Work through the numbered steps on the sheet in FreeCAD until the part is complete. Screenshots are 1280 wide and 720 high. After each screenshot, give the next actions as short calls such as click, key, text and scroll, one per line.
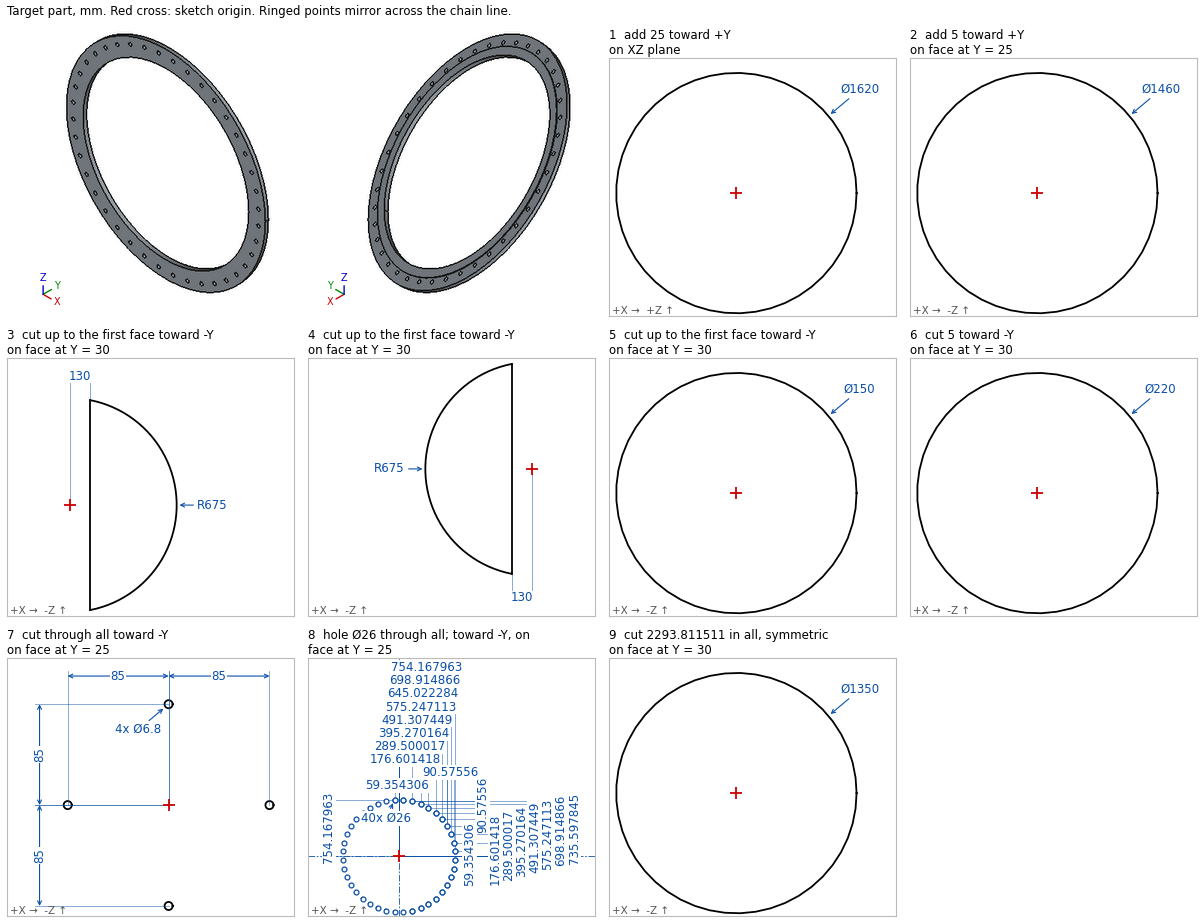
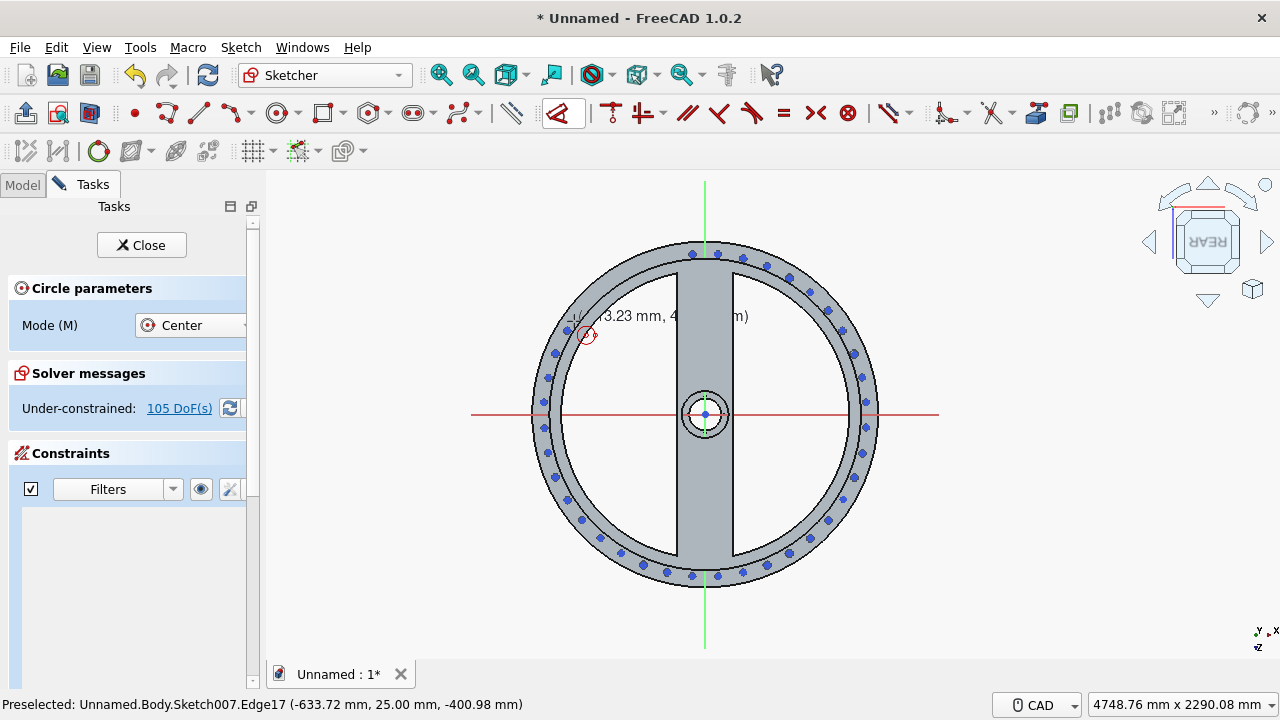
click(582, 310)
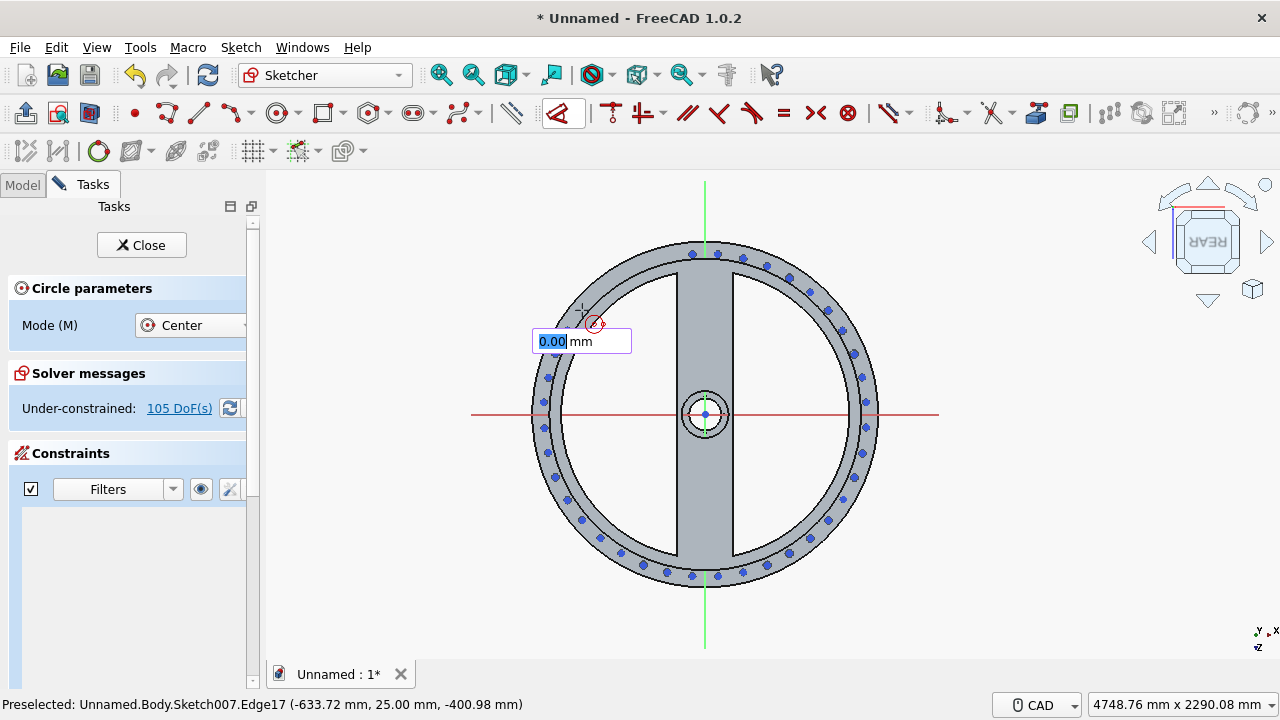
scroll(584, 308, up, 9)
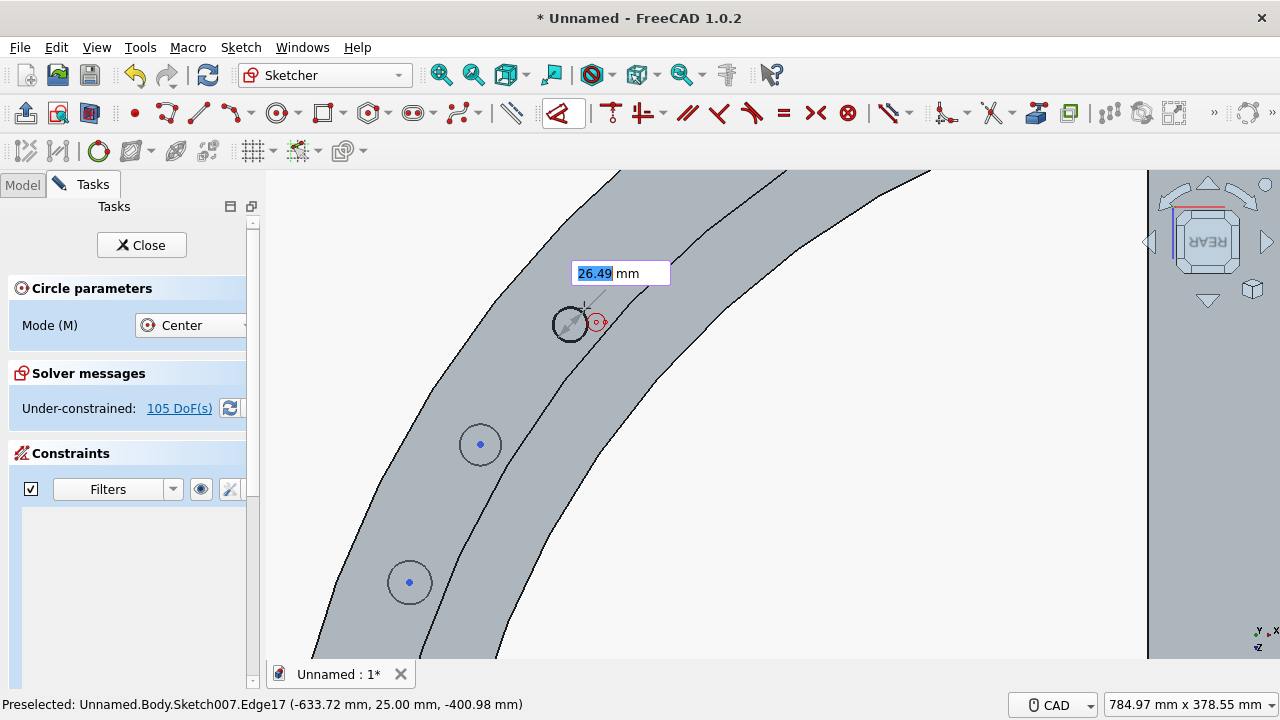
click(584, 304)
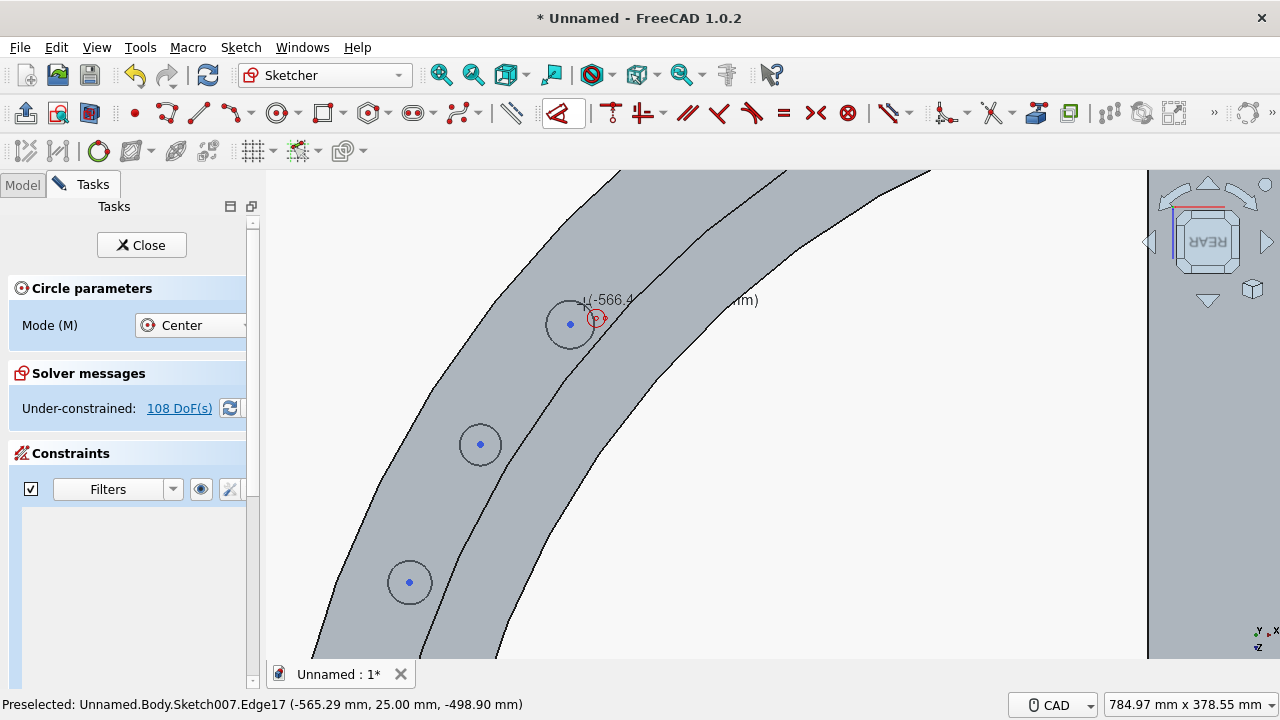
scroll(681, 208, up, 2)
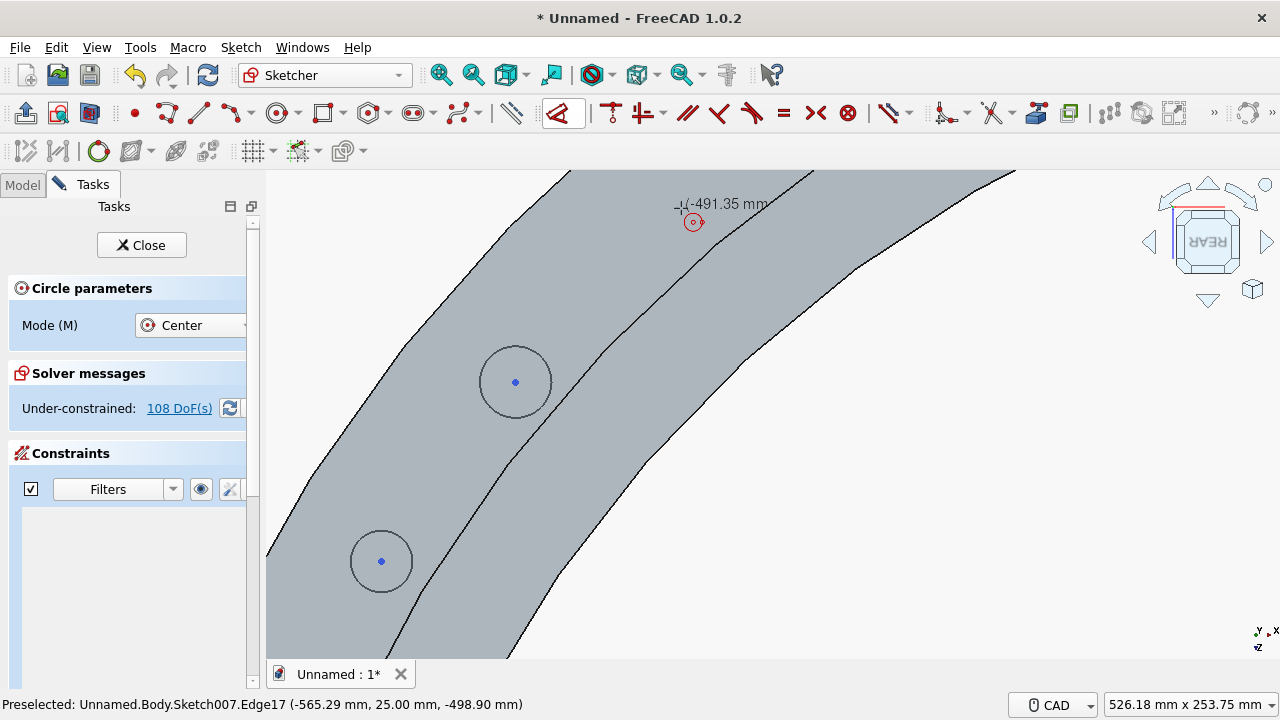
scroll(589, 302, down, 11)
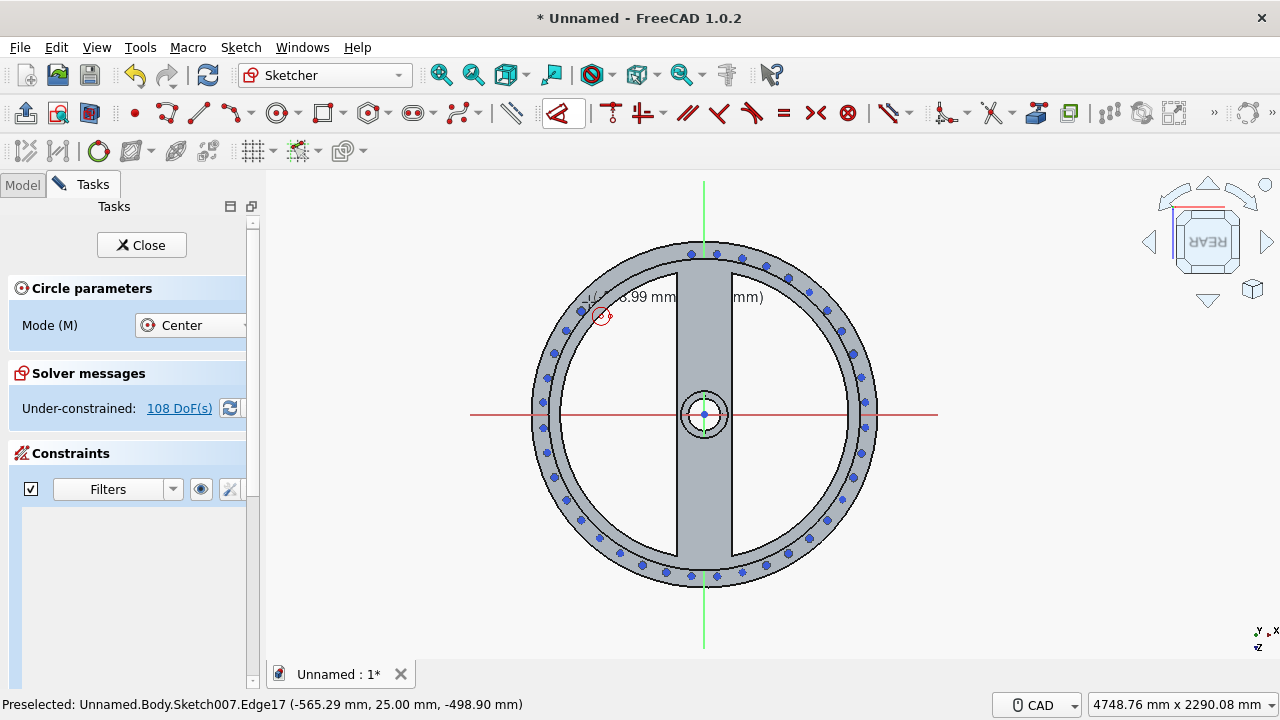
click(599, 292)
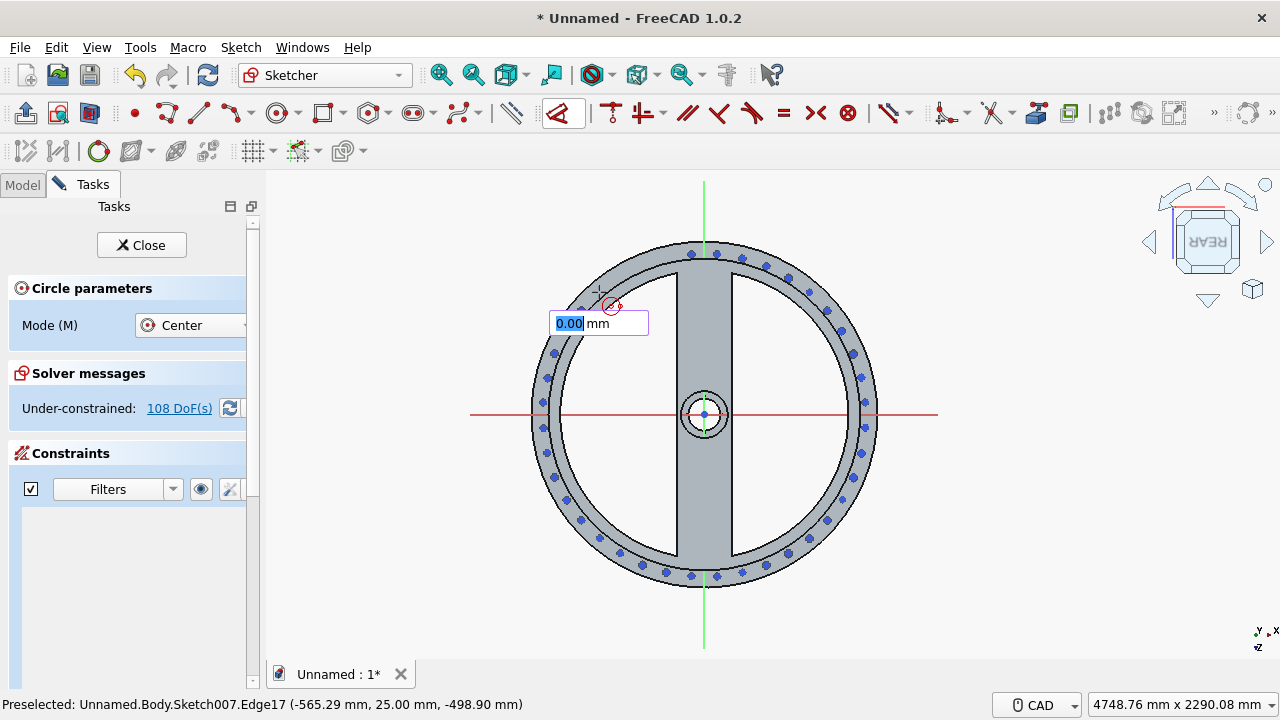
scroll(601, 290, up, 9)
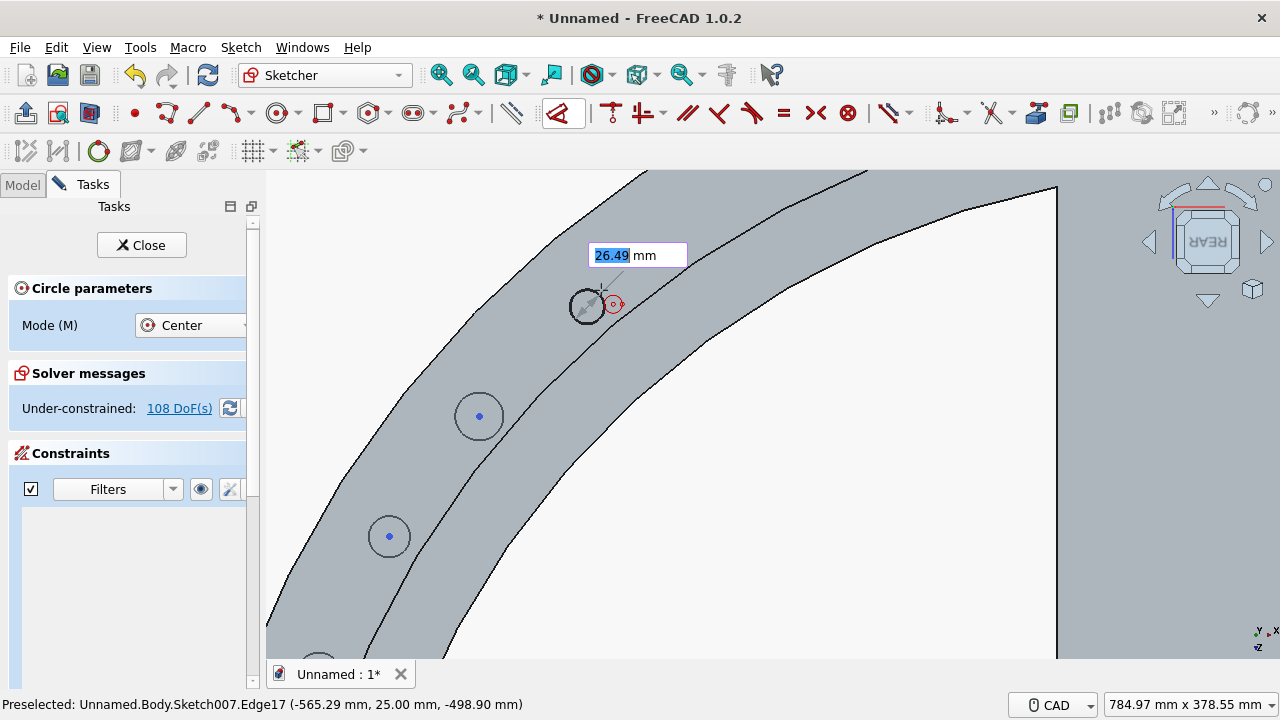
click(602, 288)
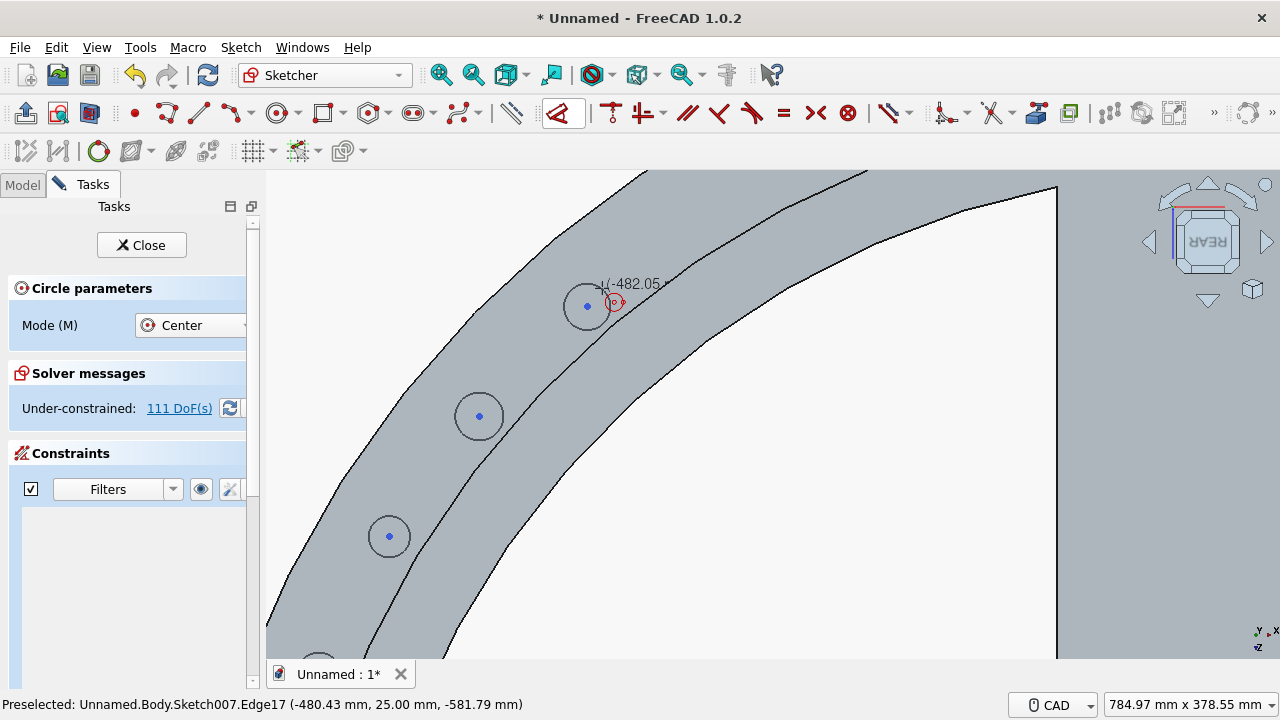
scroll(714, 209, up, 2)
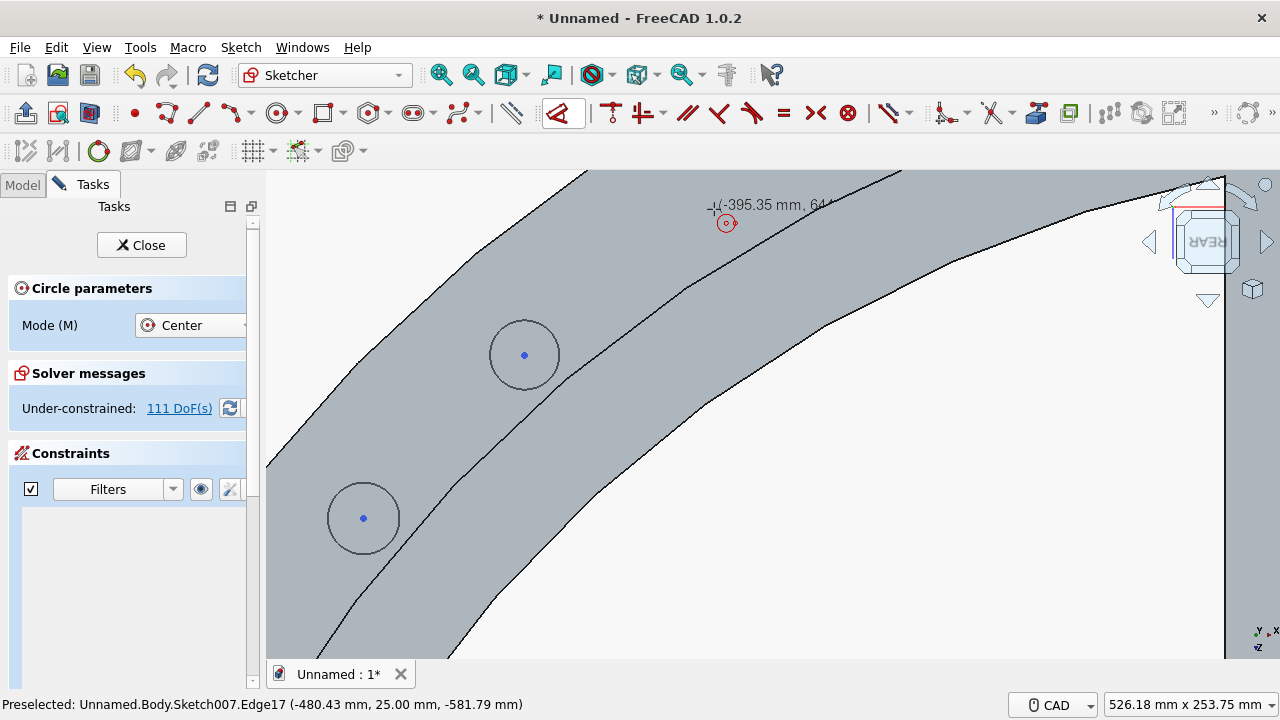
scroll(608, 285, down, 11)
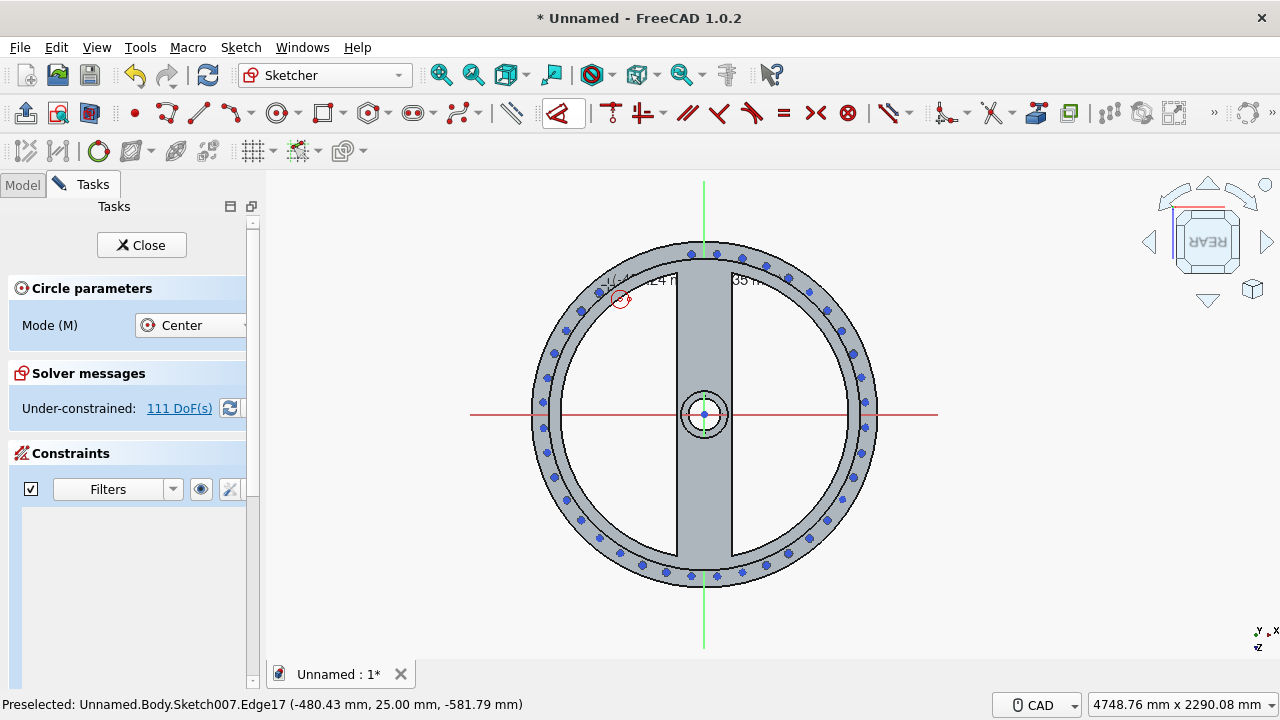
click(620, 277)